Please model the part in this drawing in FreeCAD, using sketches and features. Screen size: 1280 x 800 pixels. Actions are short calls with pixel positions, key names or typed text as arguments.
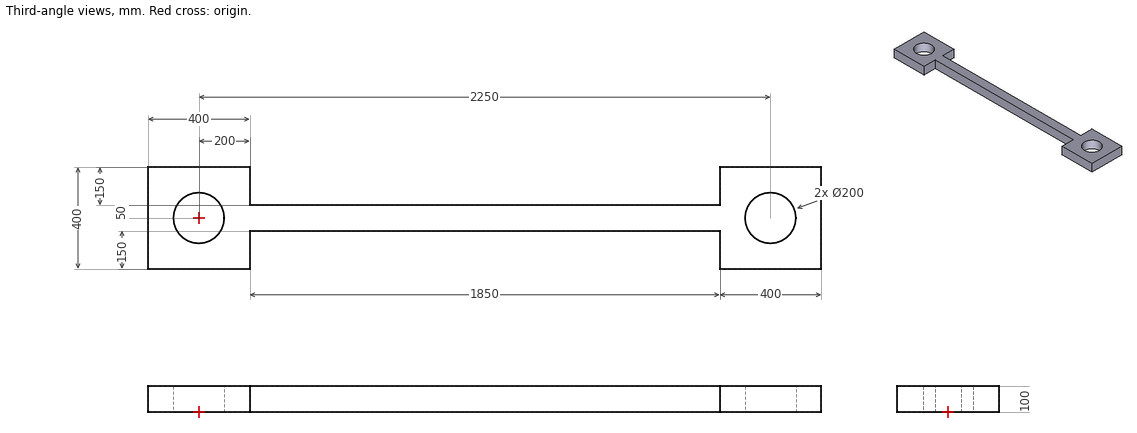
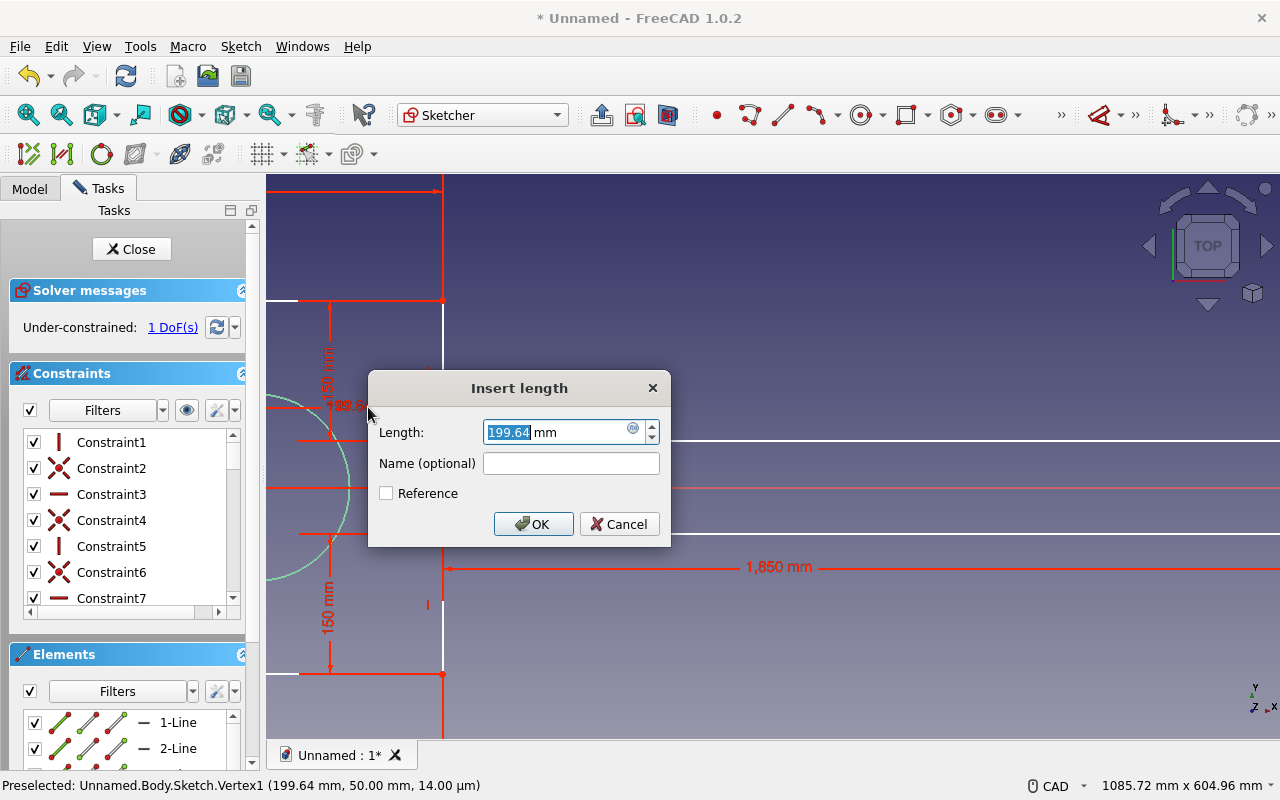
text(200)
key(Return)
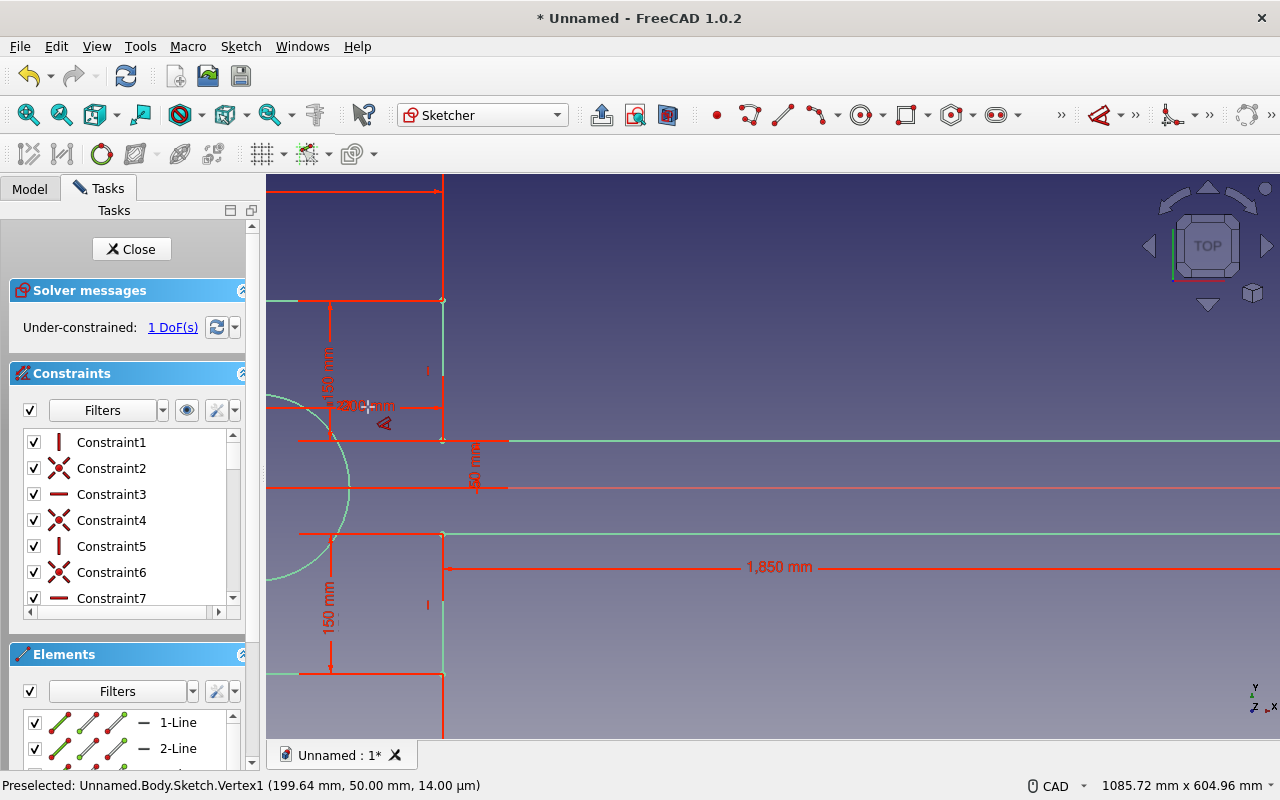
scroll(507, 446, down, 7)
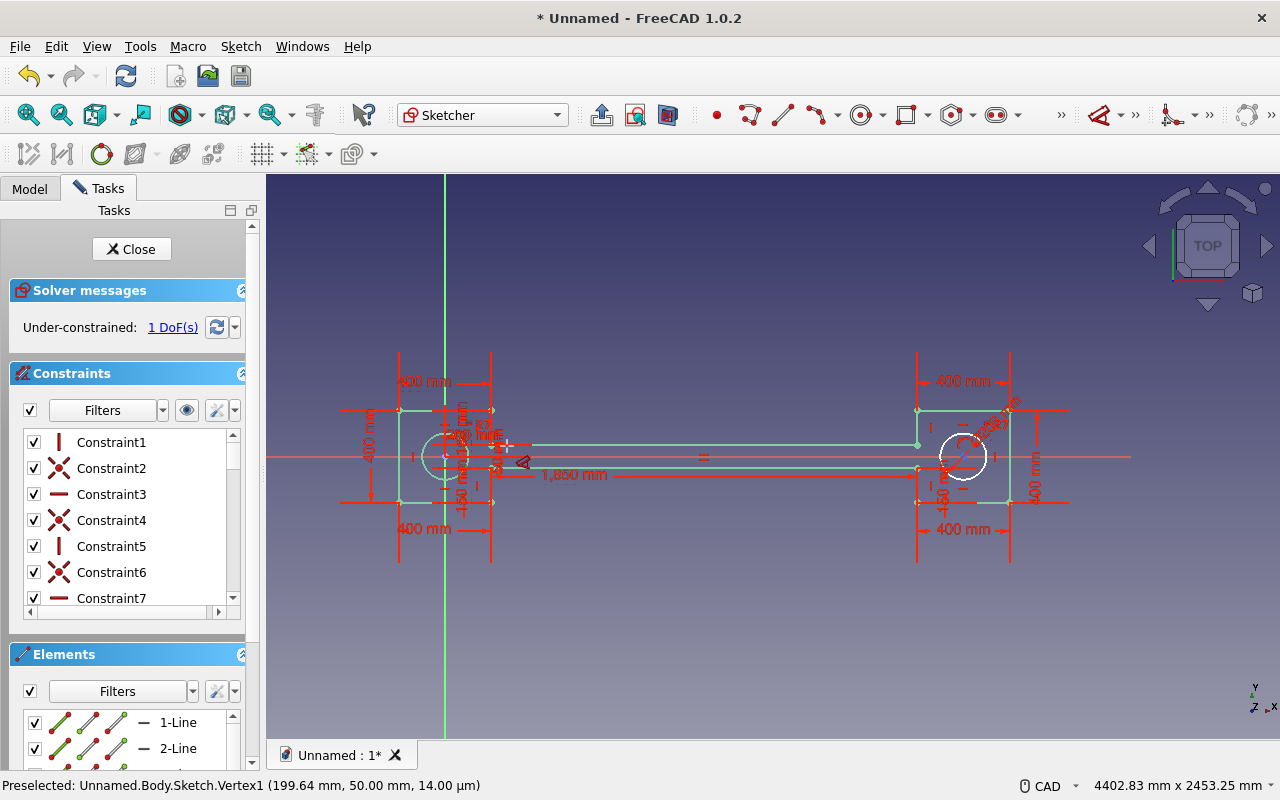
click(963, 457)
click(704, 491)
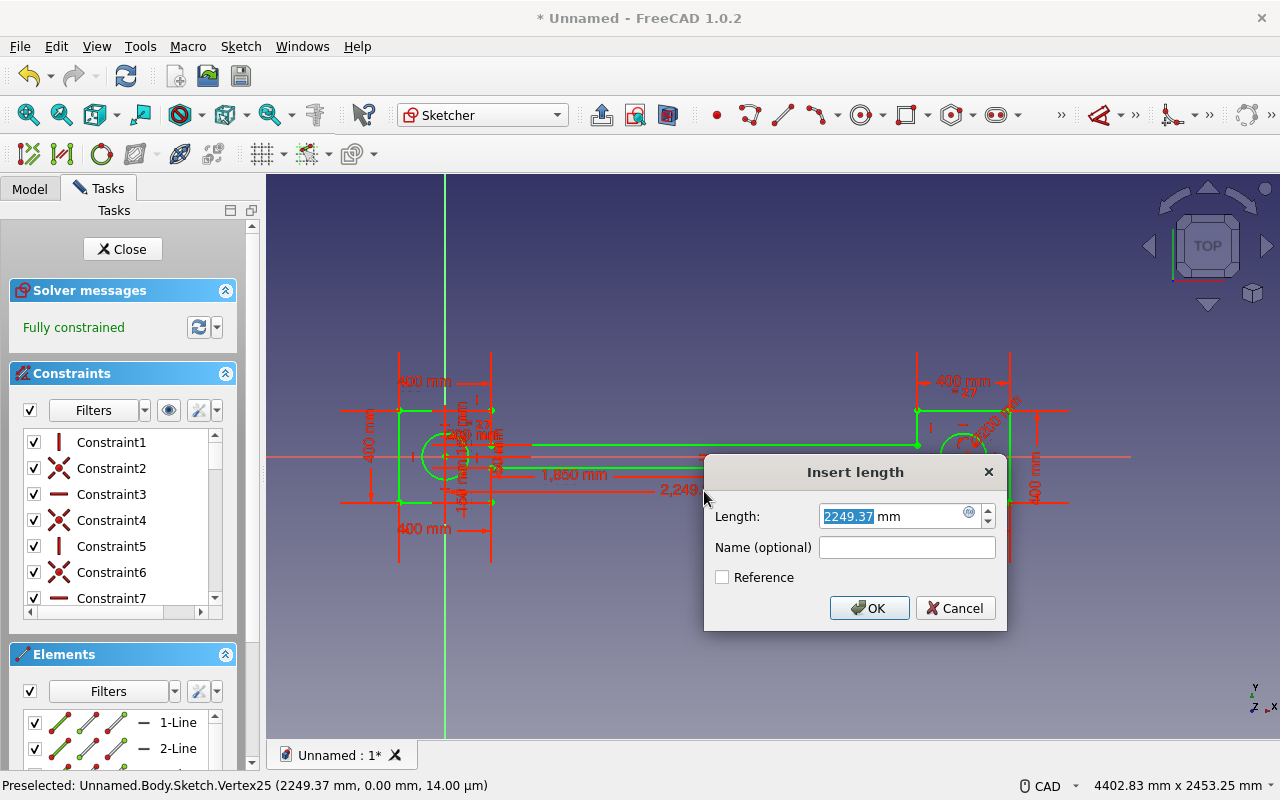
text(2250)
key(Return)
key(Escape)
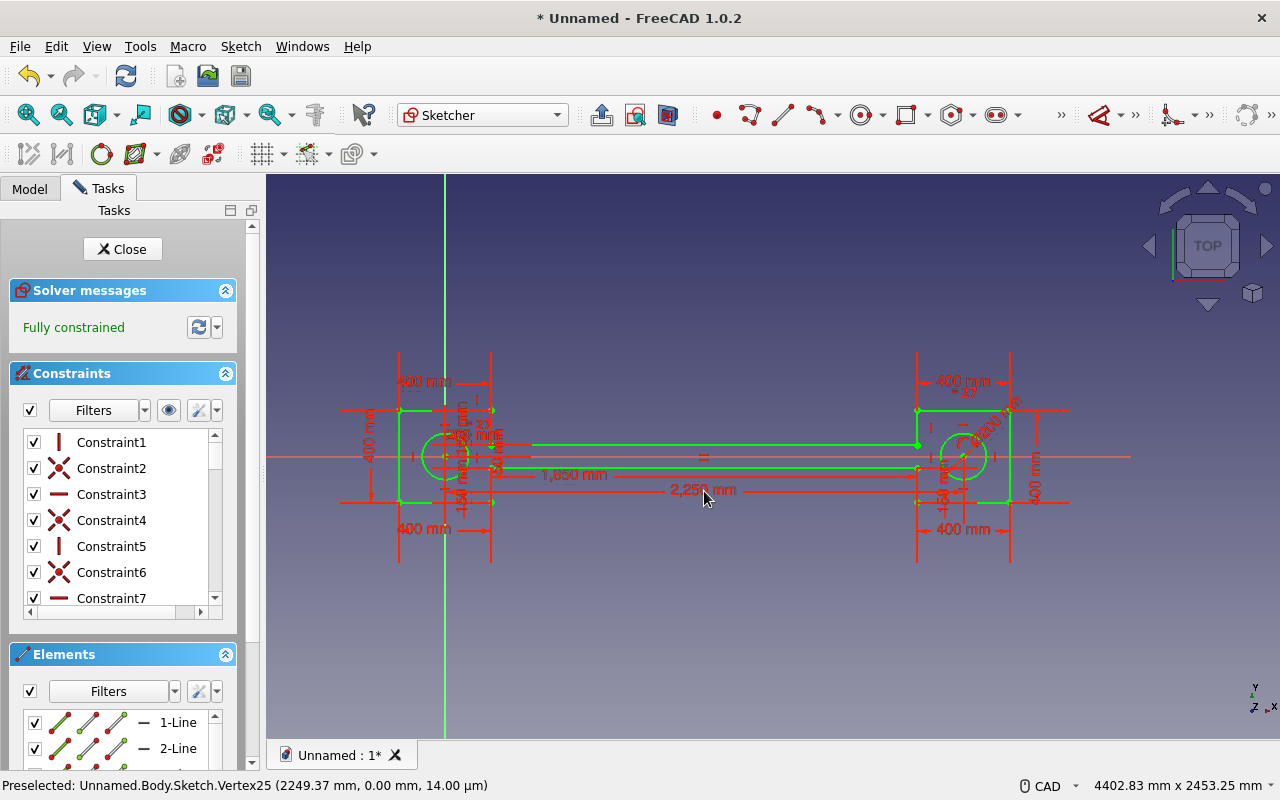
click(123, 249)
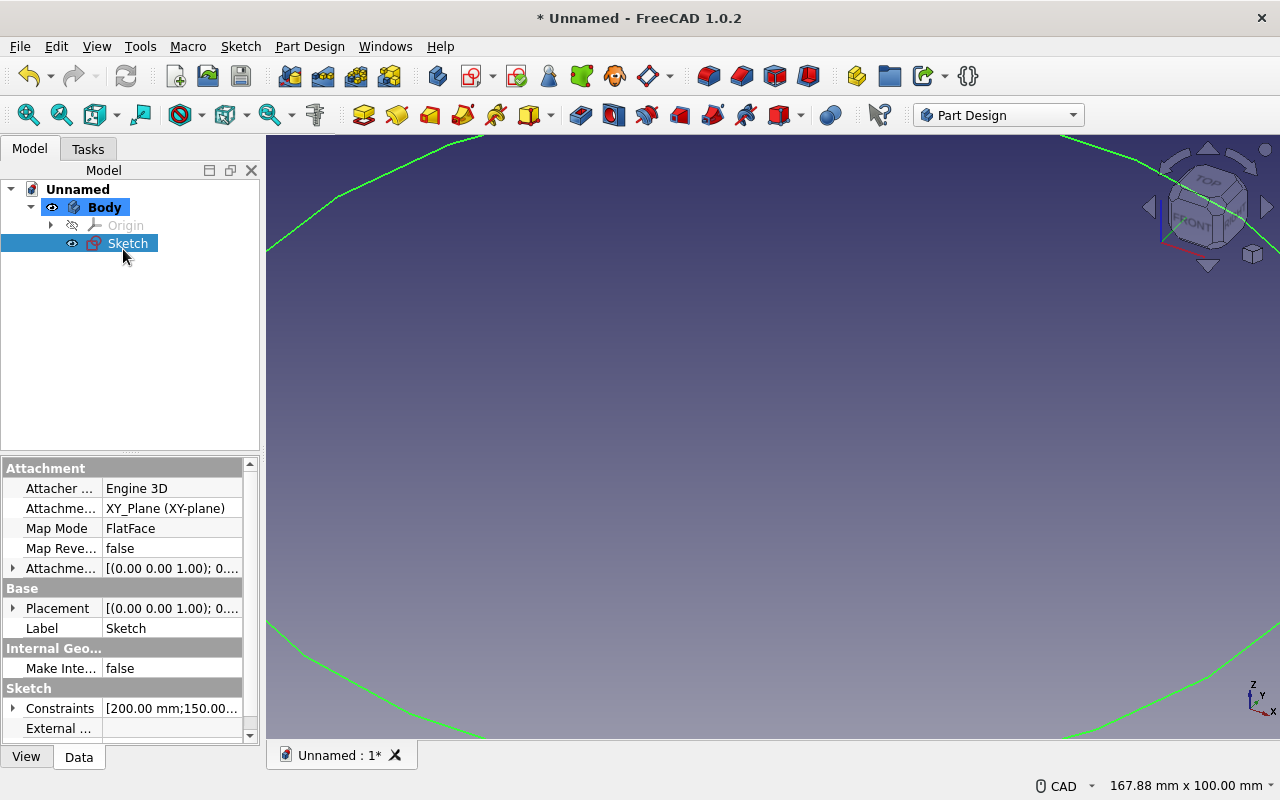
click(364, 116)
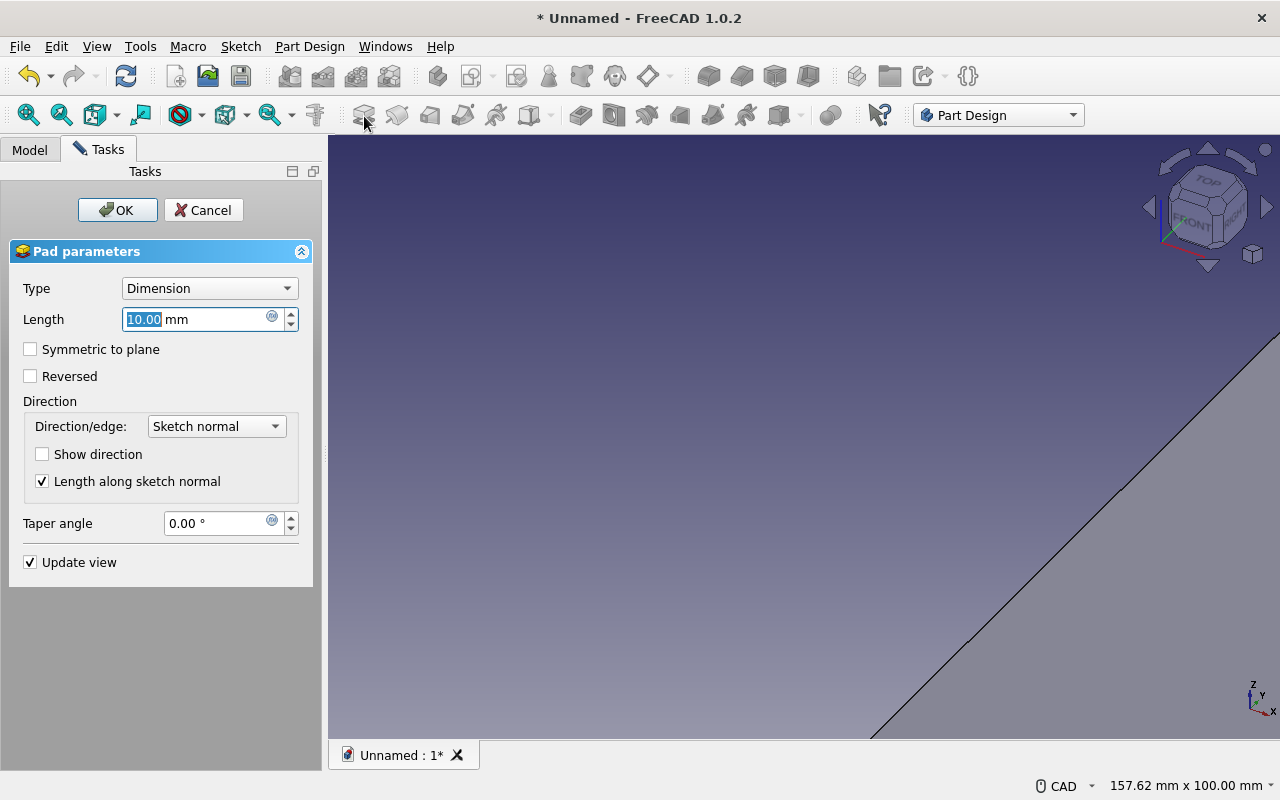
text(100)
key(Tab)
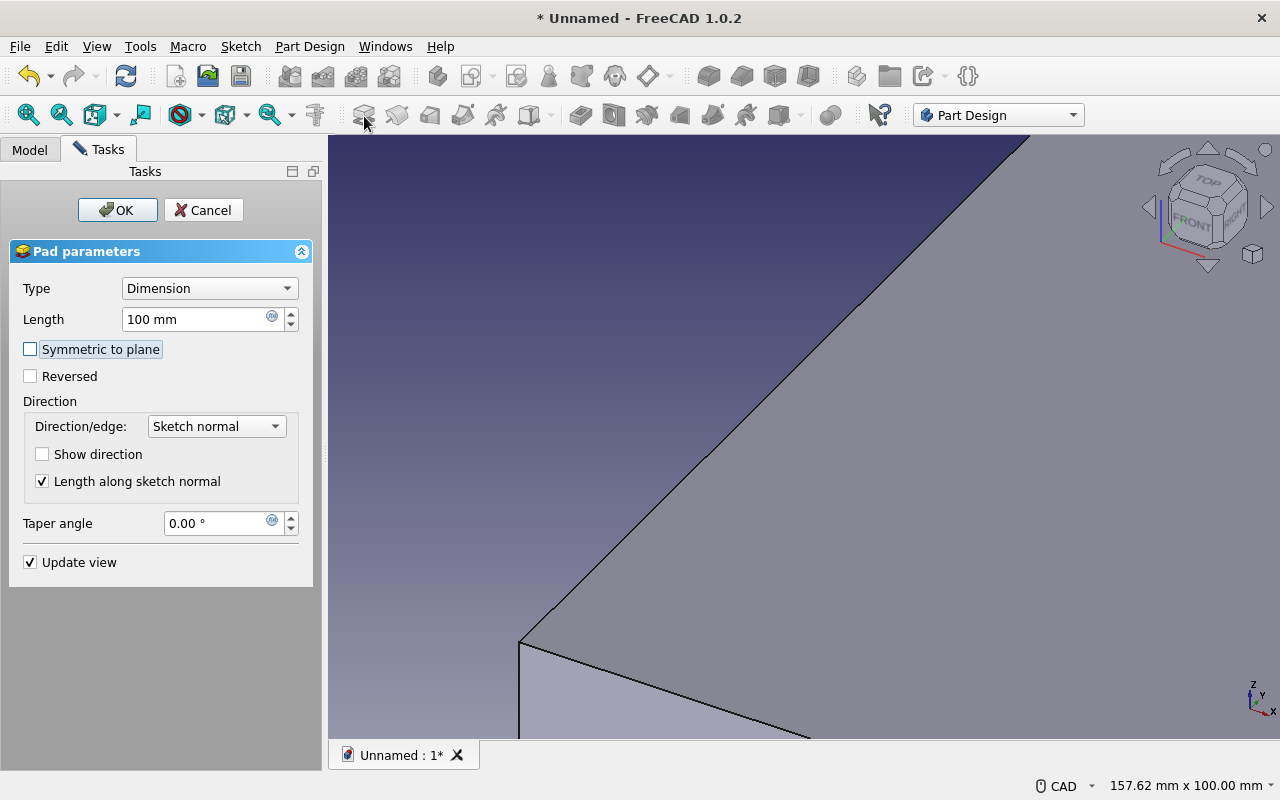
click(118, 210)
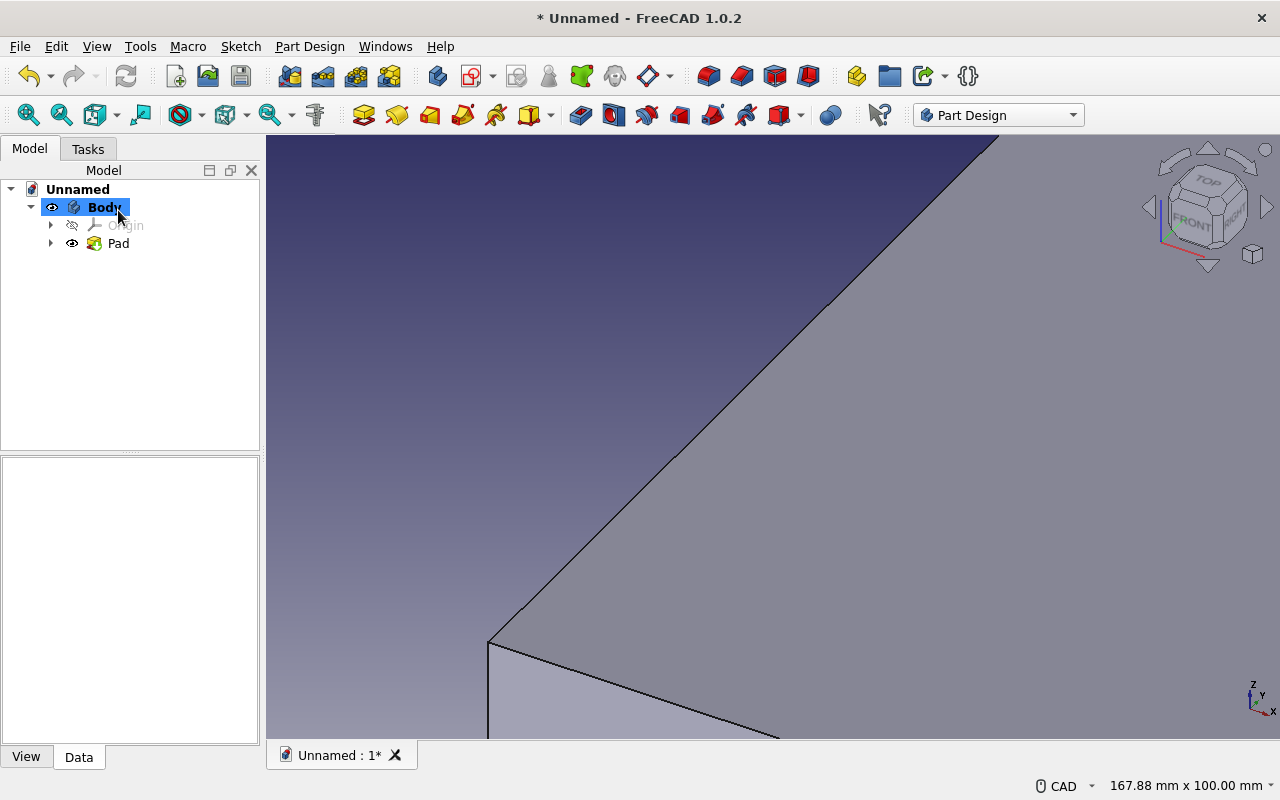
key(0)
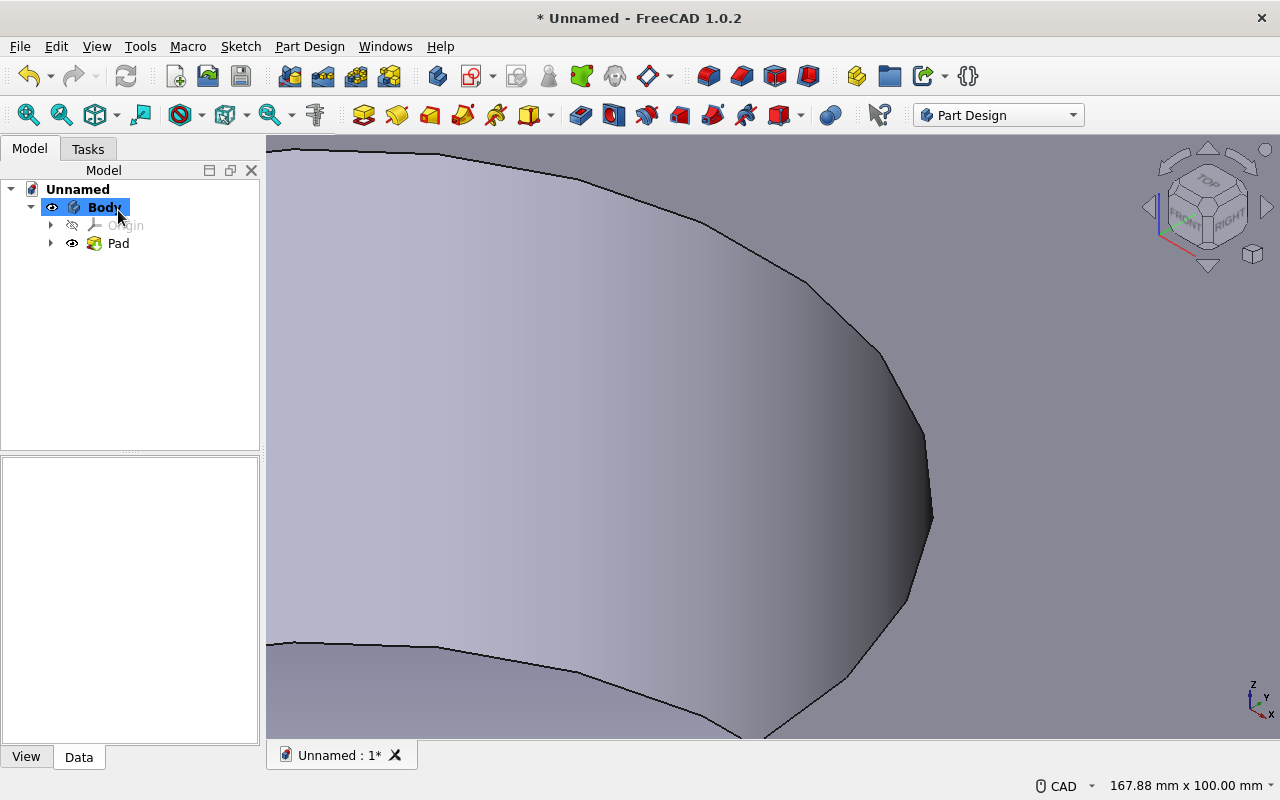
click(29, 116)